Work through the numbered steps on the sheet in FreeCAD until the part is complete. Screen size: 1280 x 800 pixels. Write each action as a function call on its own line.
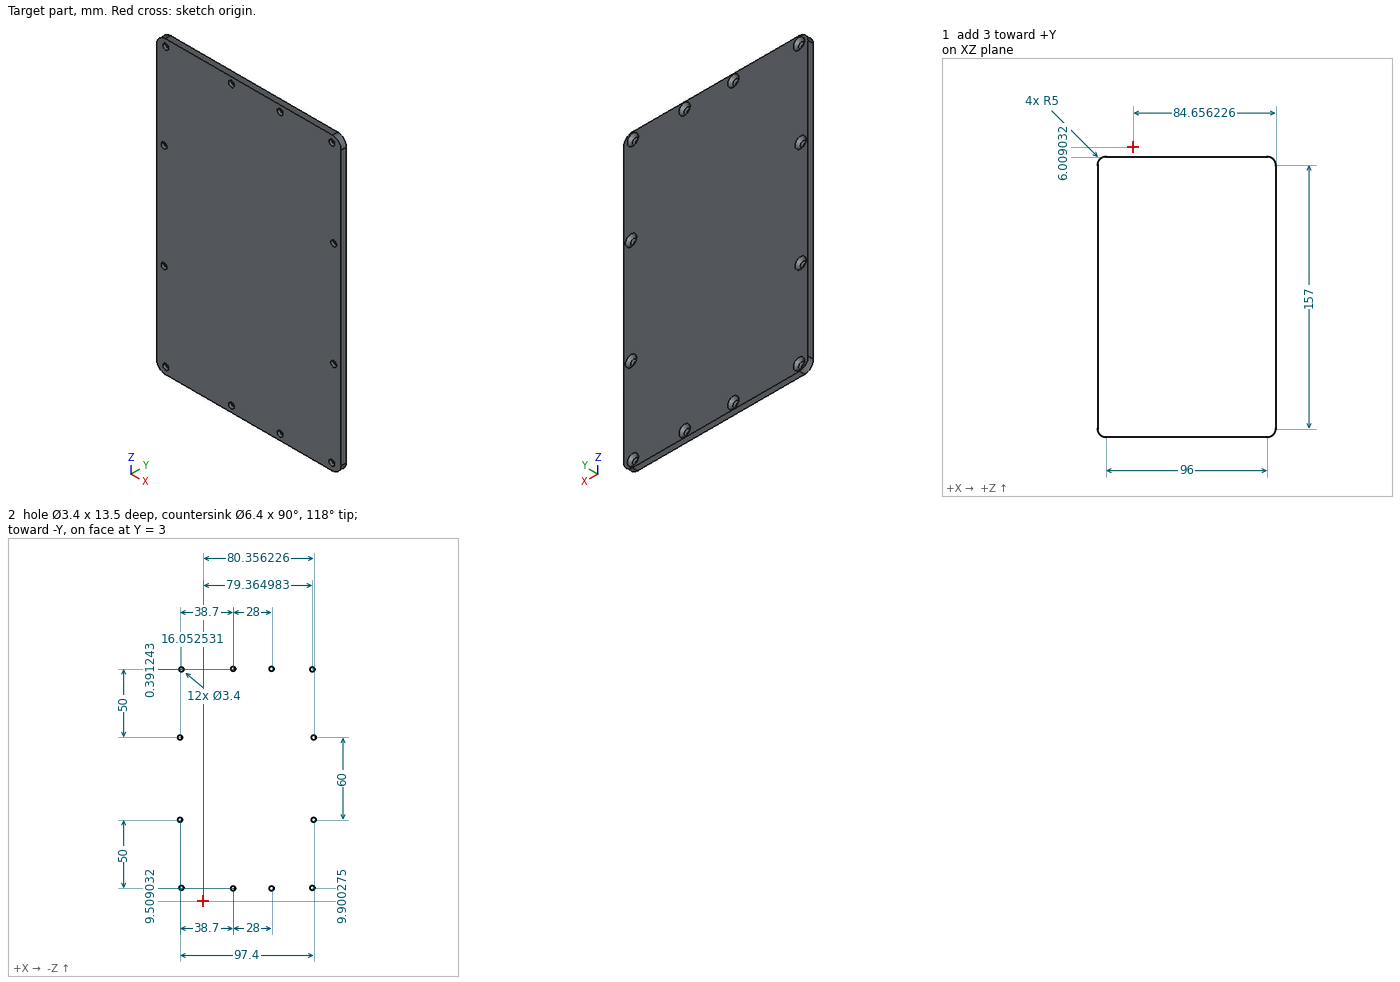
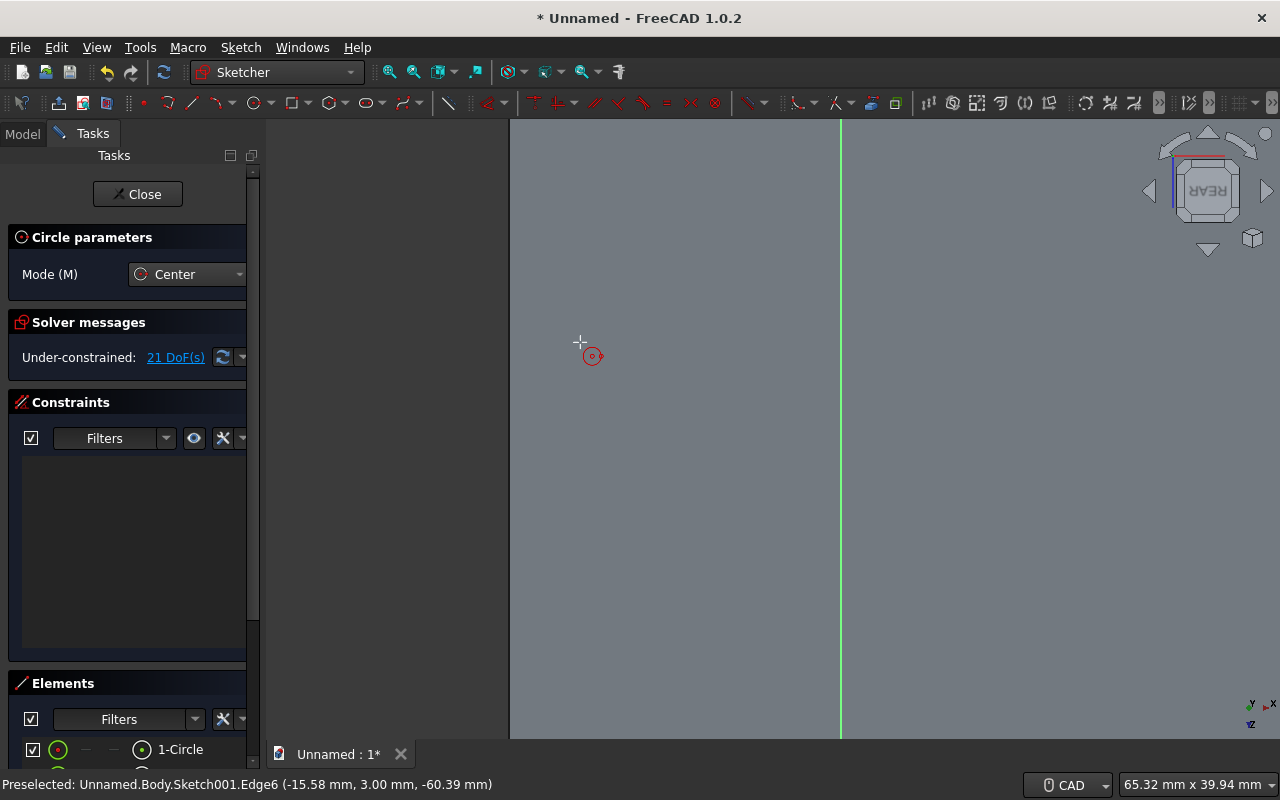
scroll(580, 342, down, 9)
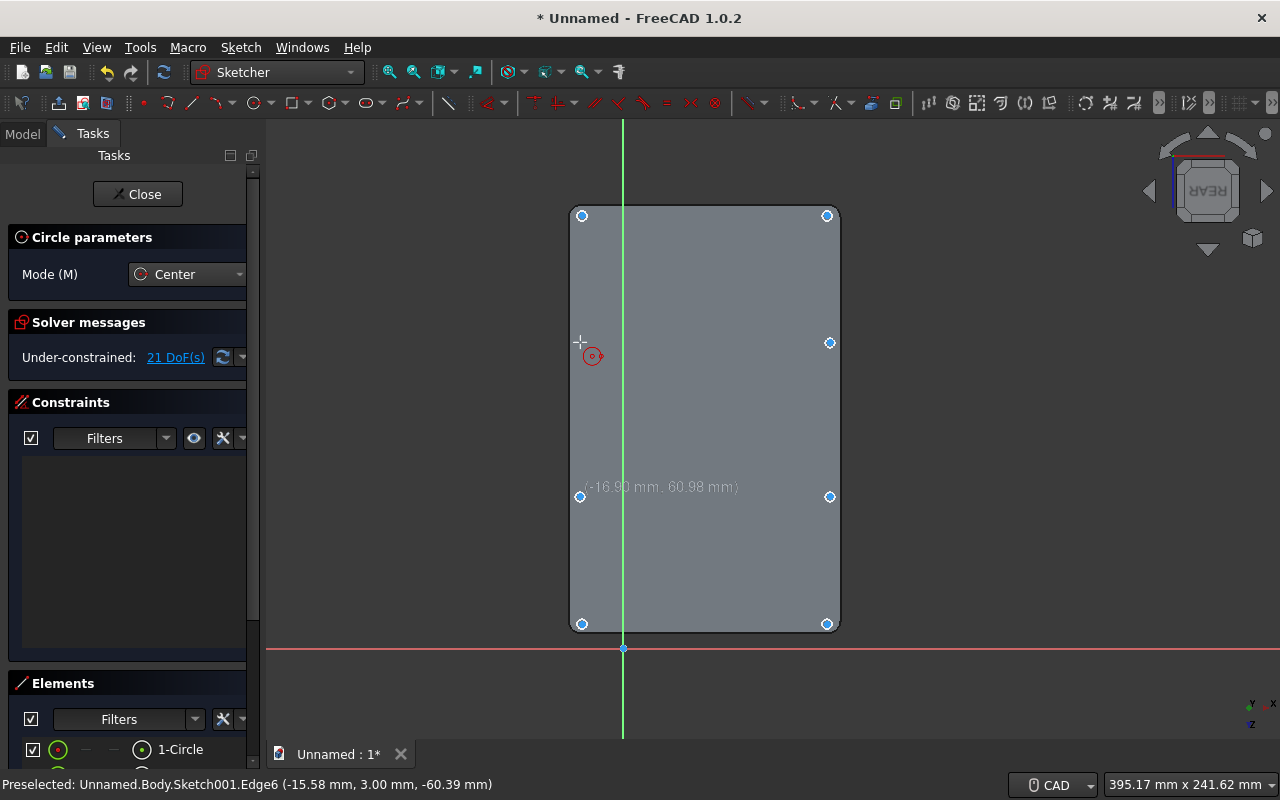
click(580, 342)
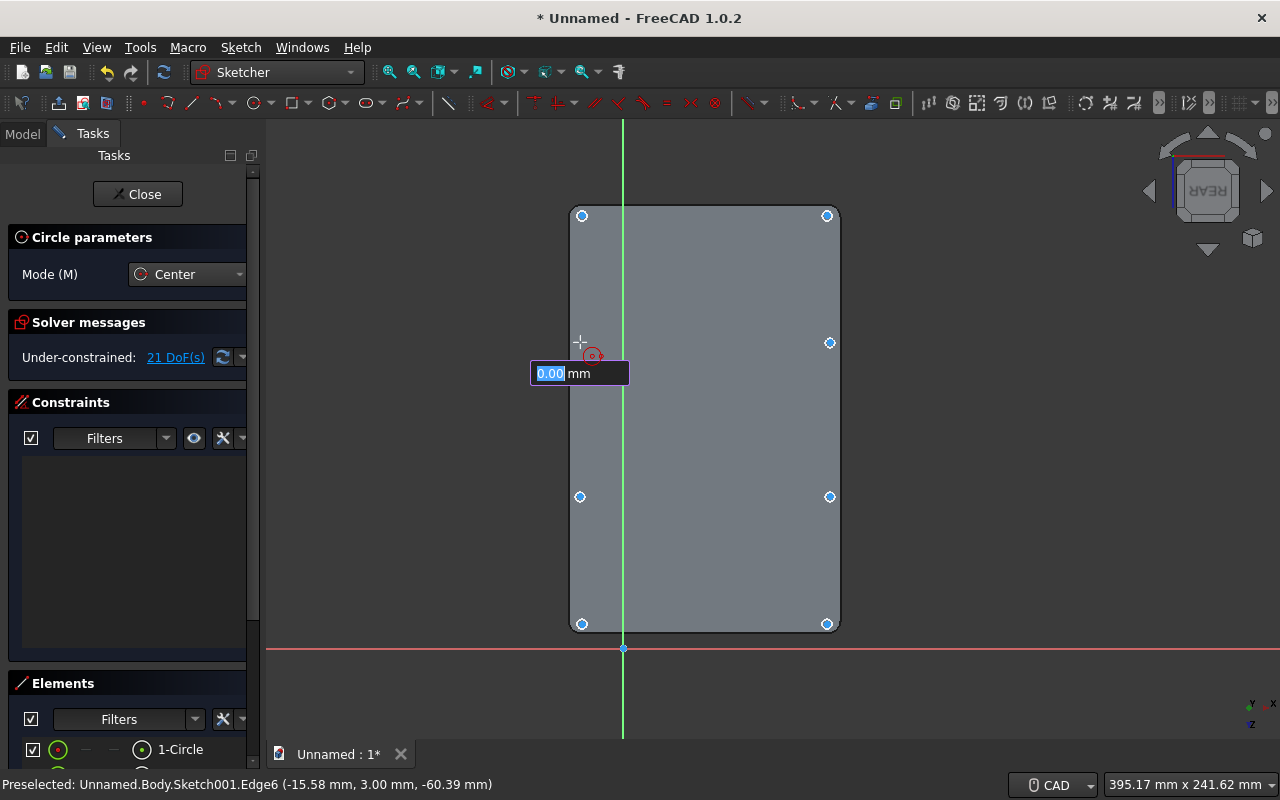
scroll(583, 339, up, 7)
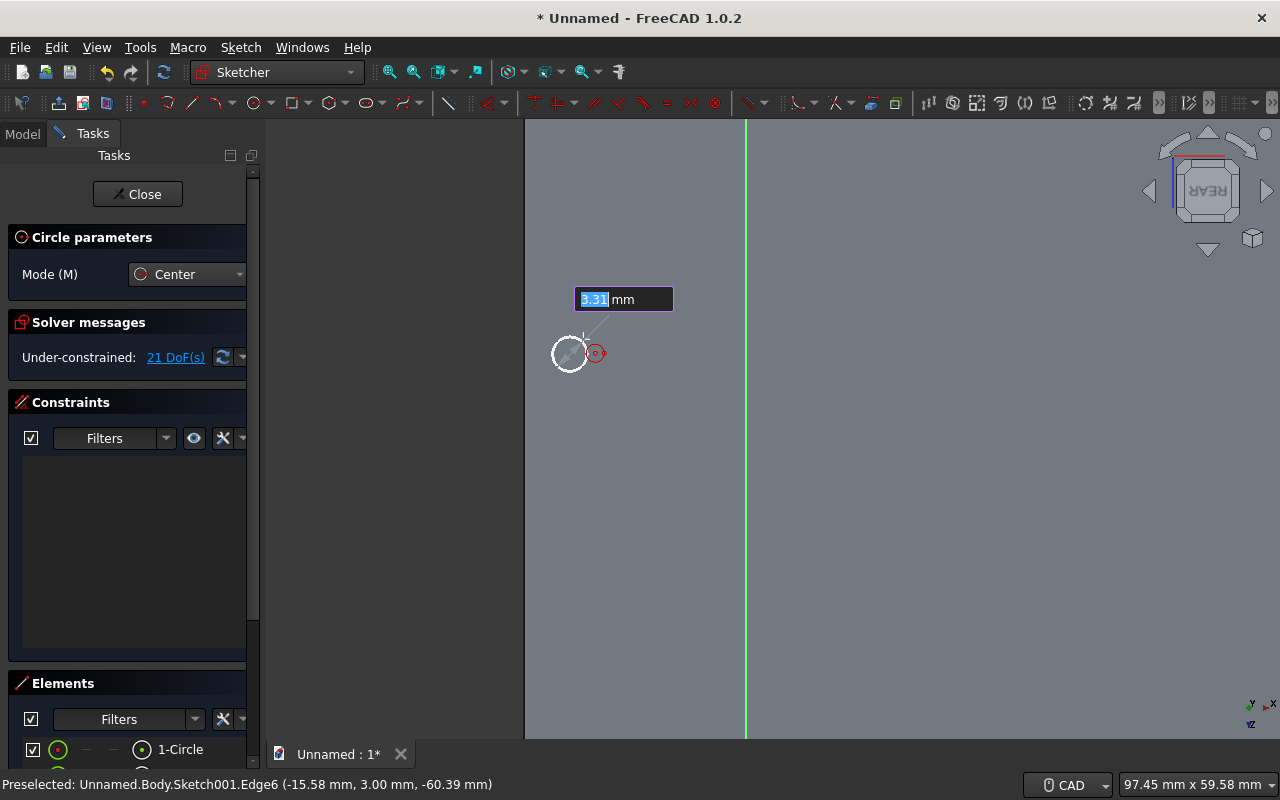
click(581, 338)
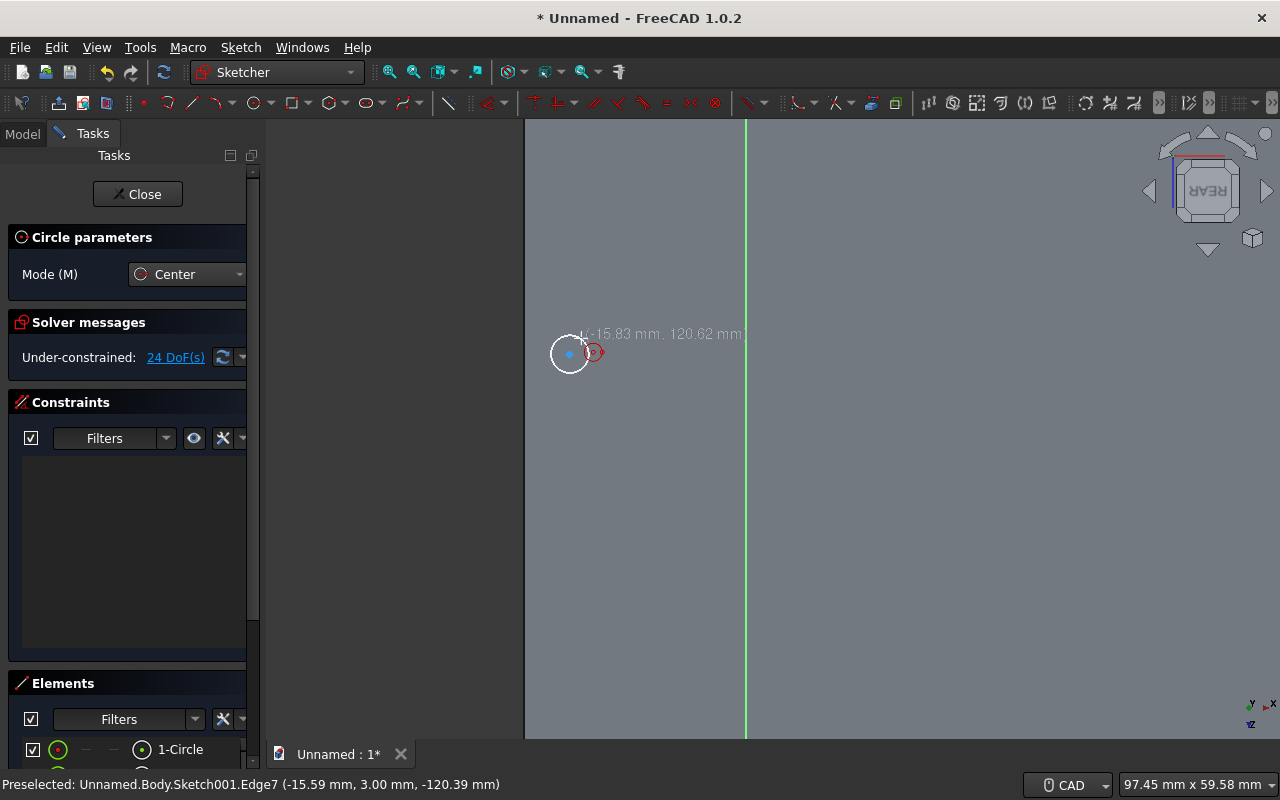
scroll(583, 339, down, 7)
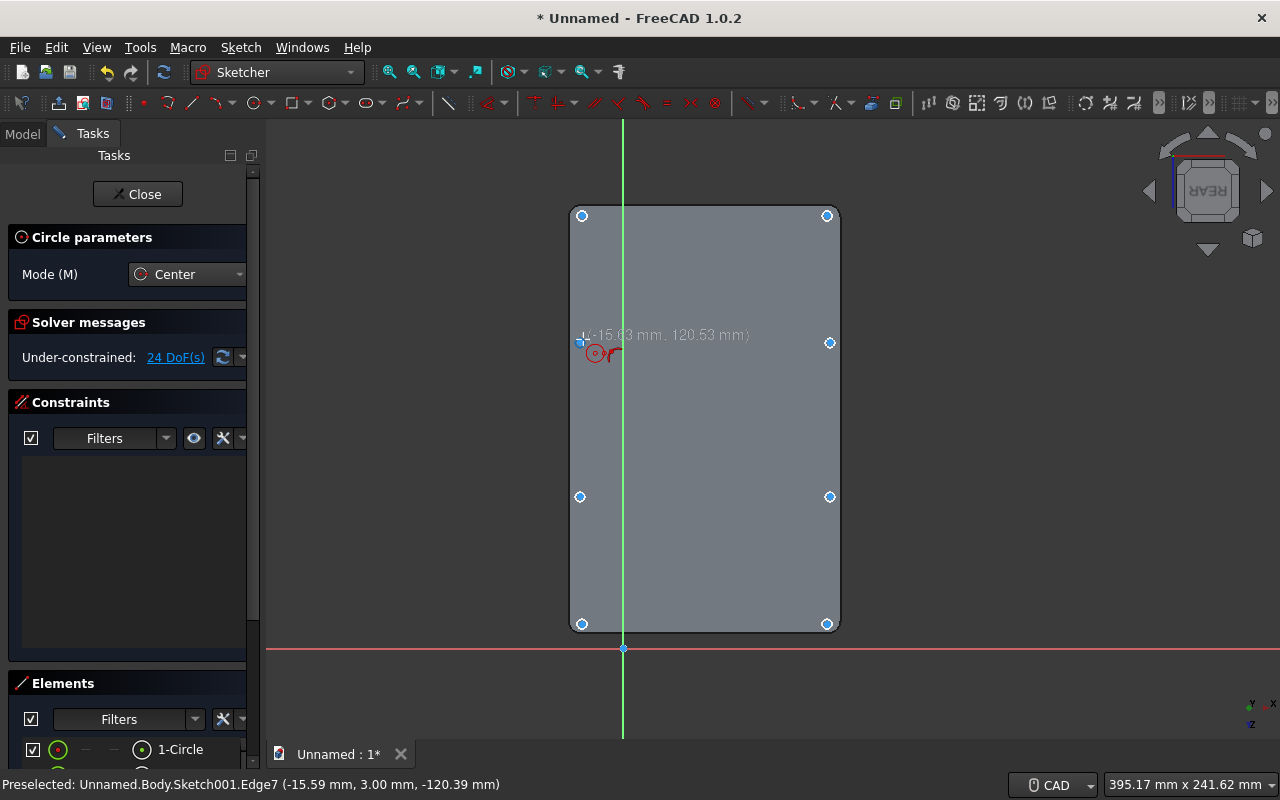
scroll(679, 214, up, 9)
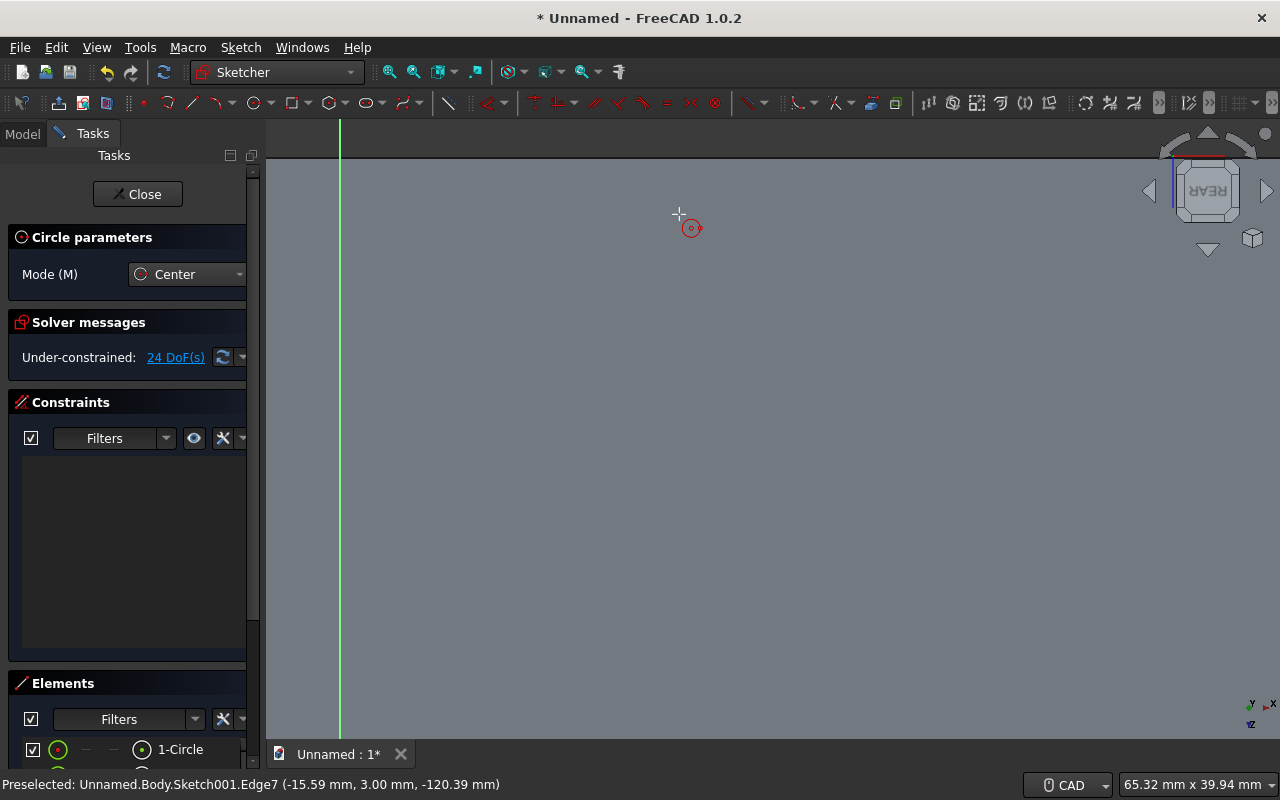
scroll(679, 214, down, 9)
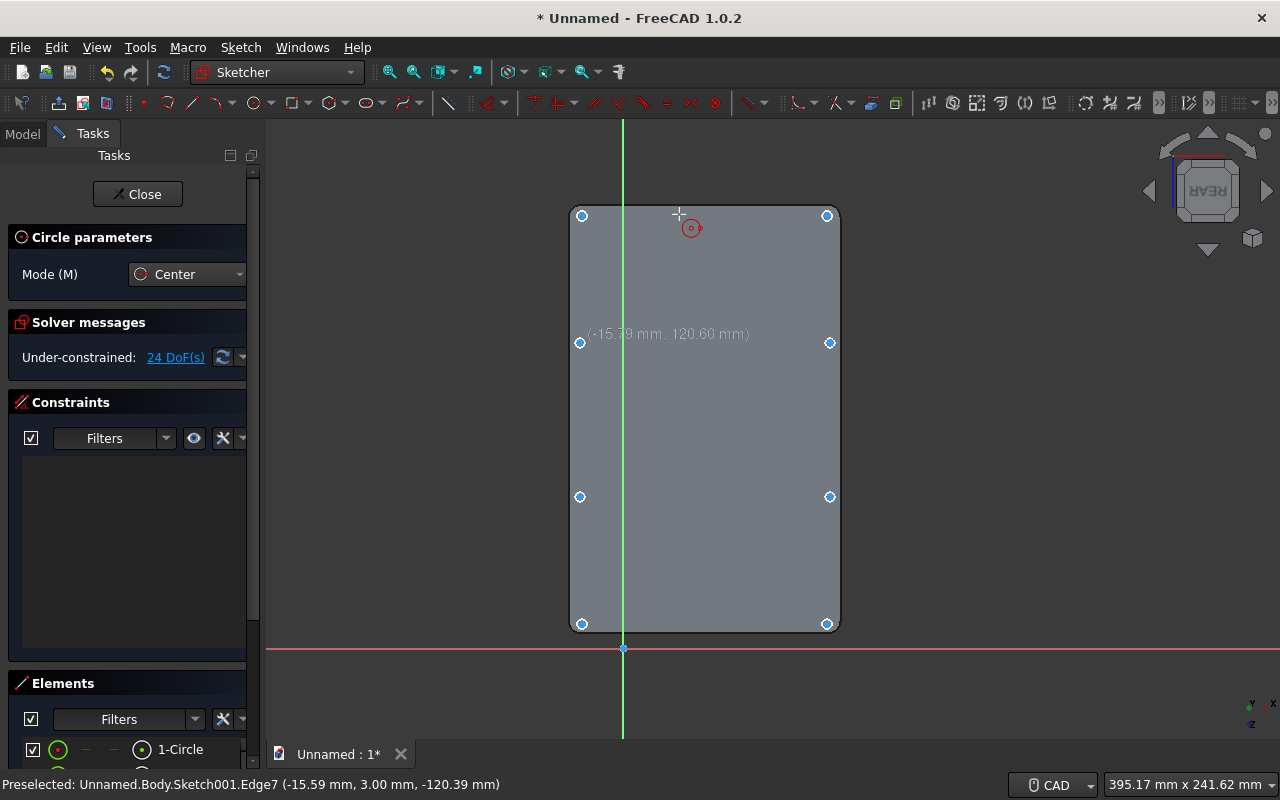
click(679, 214)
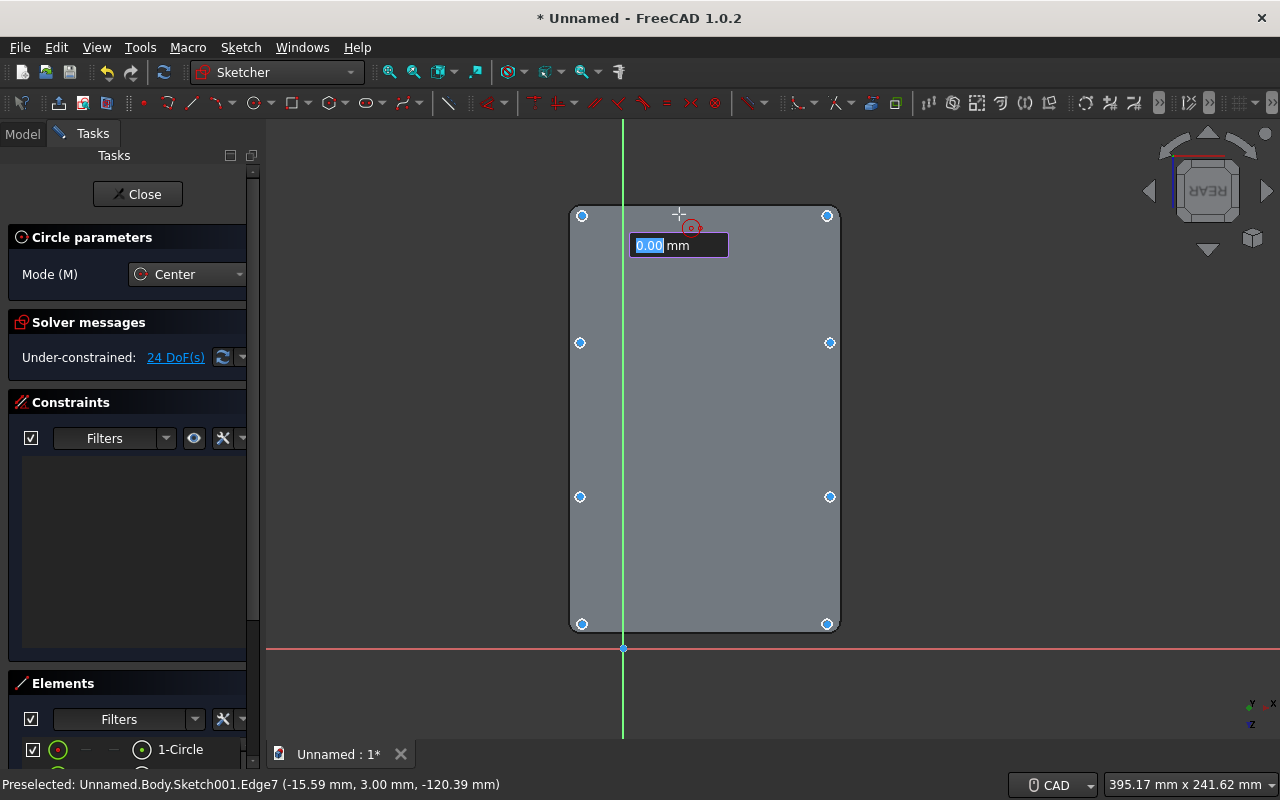
scroll(682, 211, up, 7)